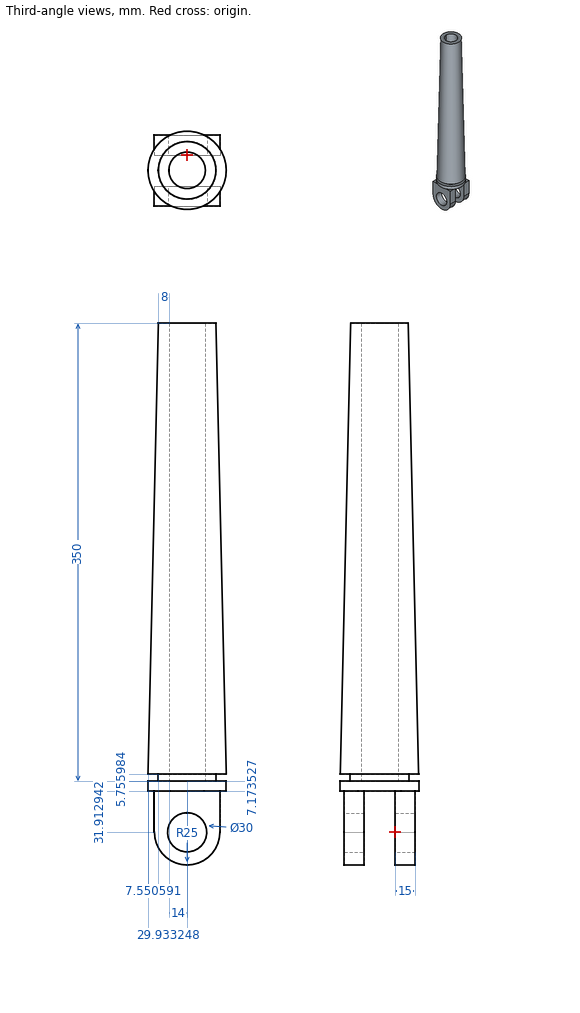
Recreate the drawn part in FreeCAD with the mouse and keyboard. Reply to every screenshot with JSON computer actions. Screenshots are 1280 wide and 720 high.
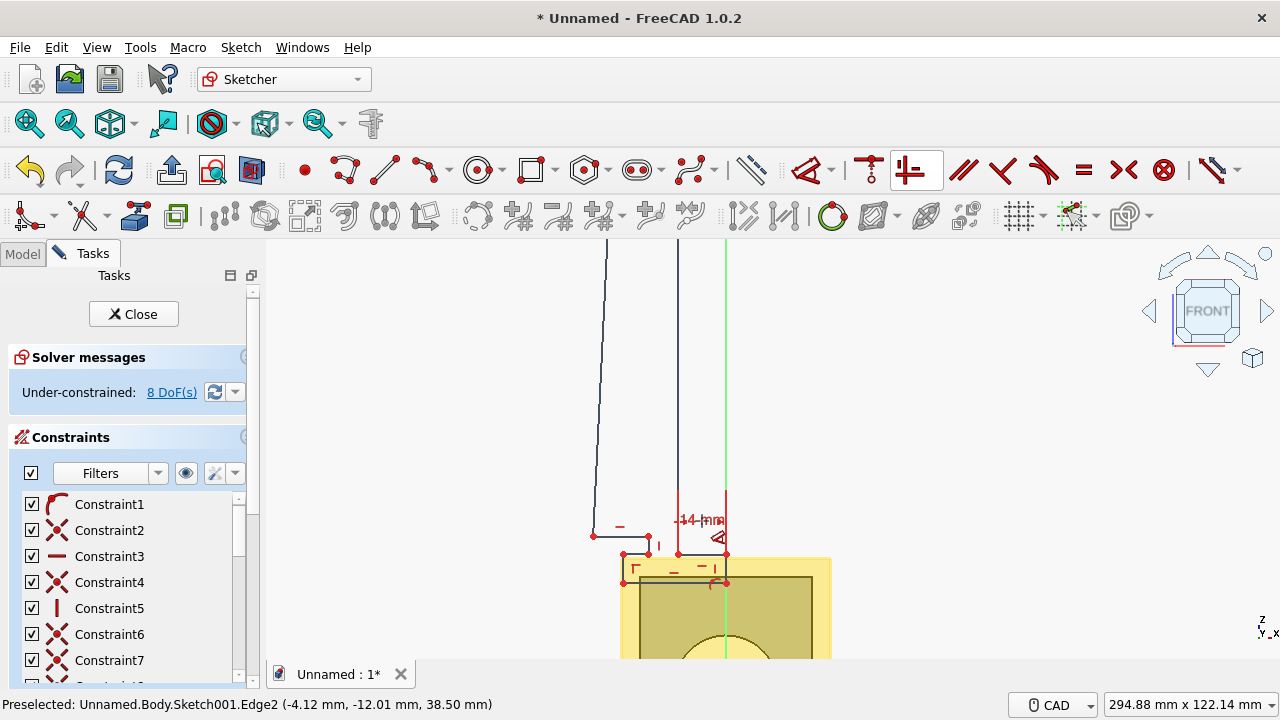
{"action": "scroll", "coordinate": [712, 558], "scroll_direction": "down", "scroll_amount": 8}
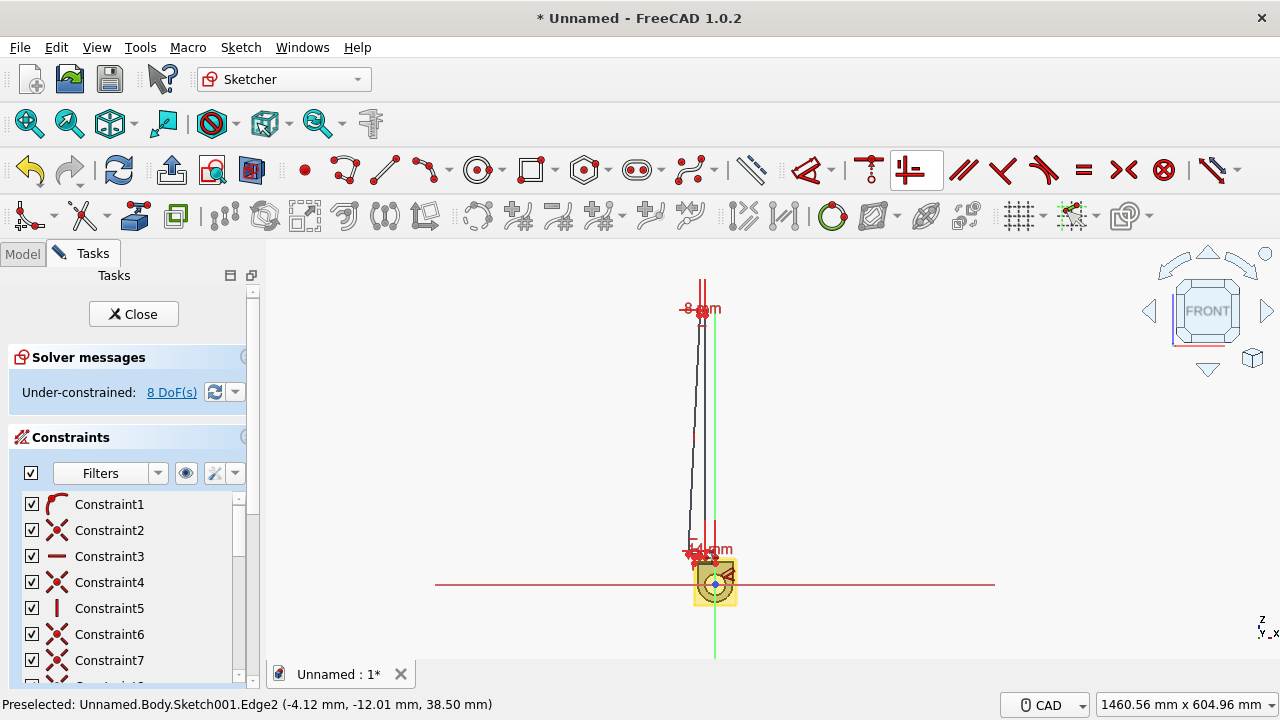
{"action": "scroll", "coordinate": [705, 509], "scroll_direction": "up", "scroll_amount": 2}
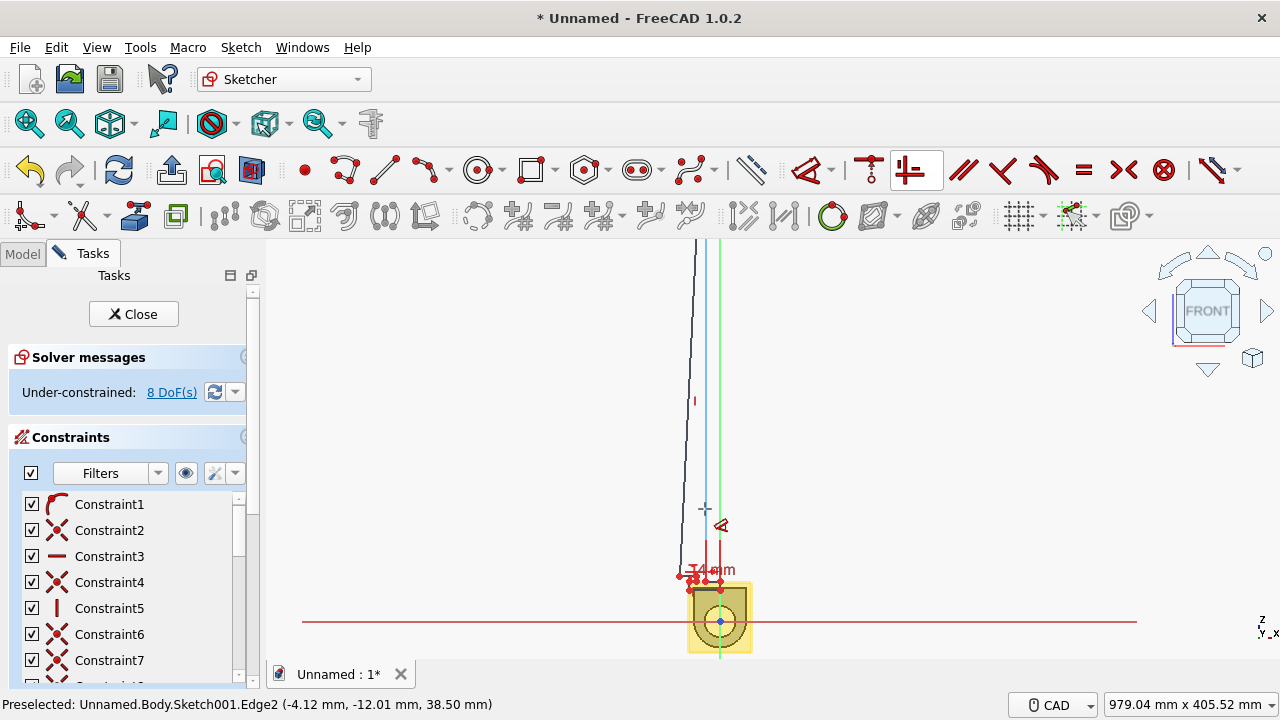
{"action": "left_click", "coordinate": [706, 509]}
{"action": "left_click", "coordinate": [740, 424]}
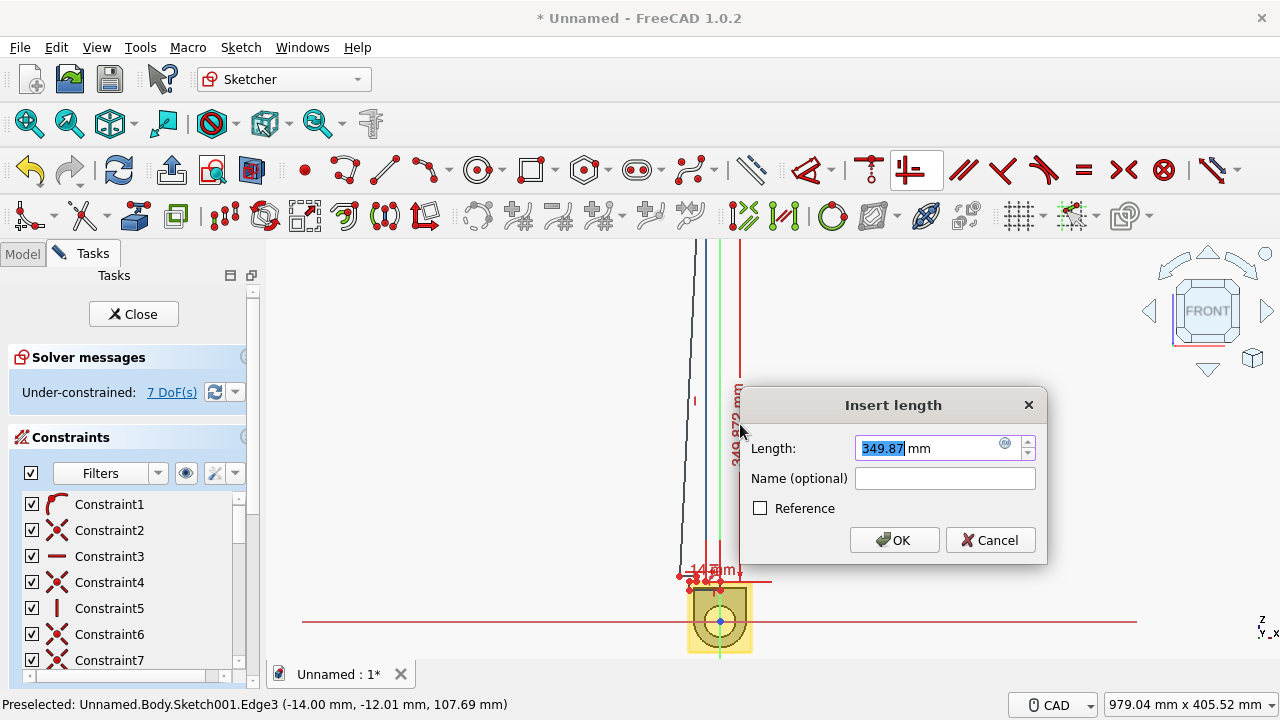
{"action": "type", "text": "350"}
{"action": "key", "text": "Return"}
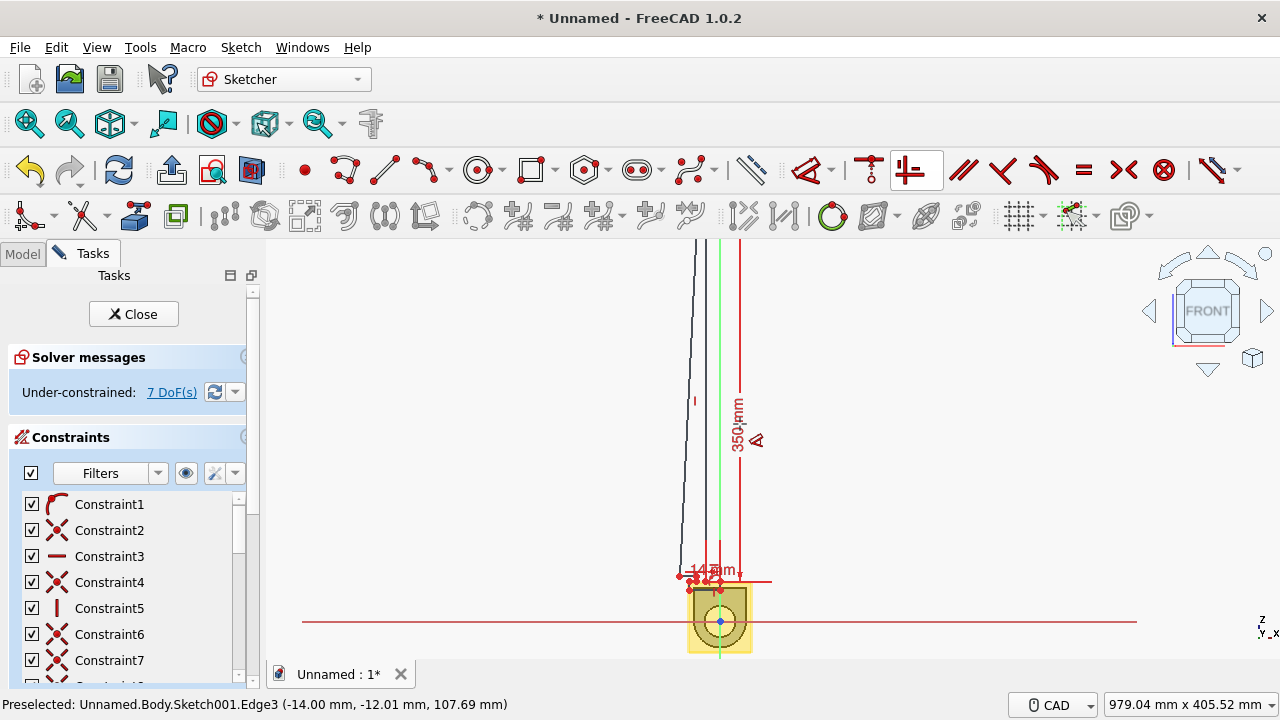
{"action": "scroll", "coordinate": [720, 586], "scroll_direction": "up", "scroll_amount": 9}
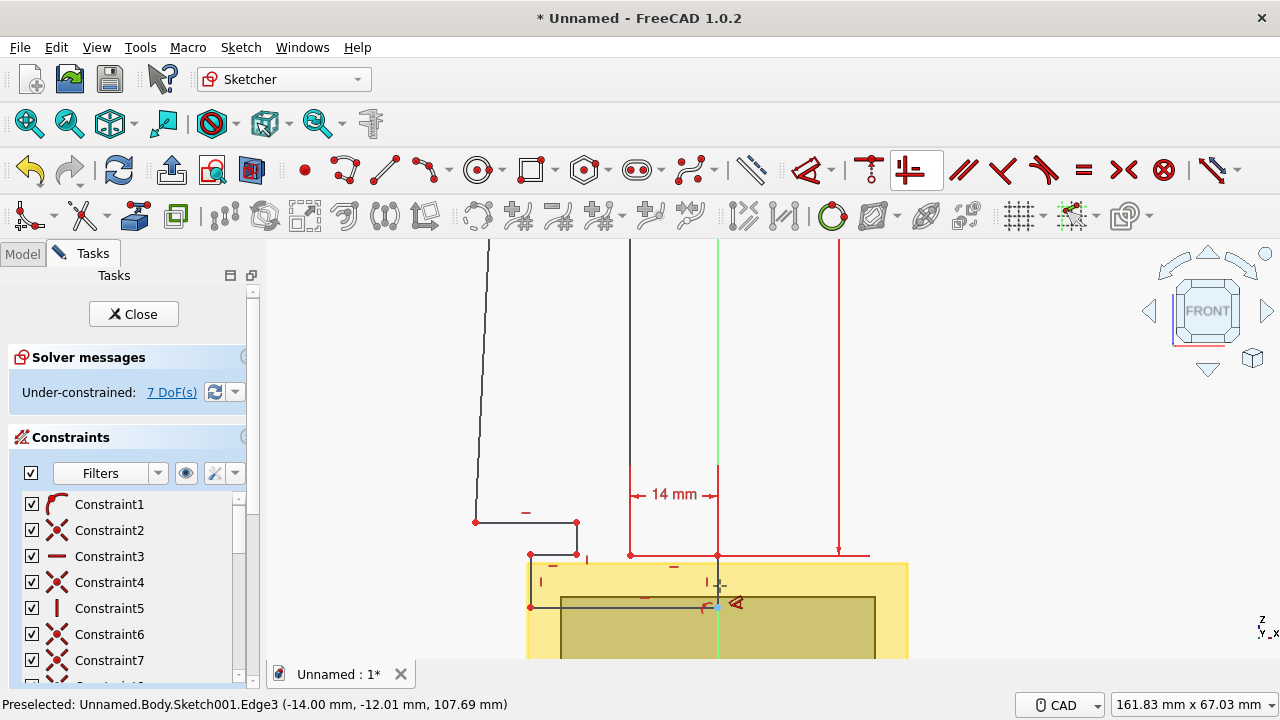
{"action": "left_click", "coordinate": [718, 582]}
{"action": "left_click", "coordinate": [752, 582]}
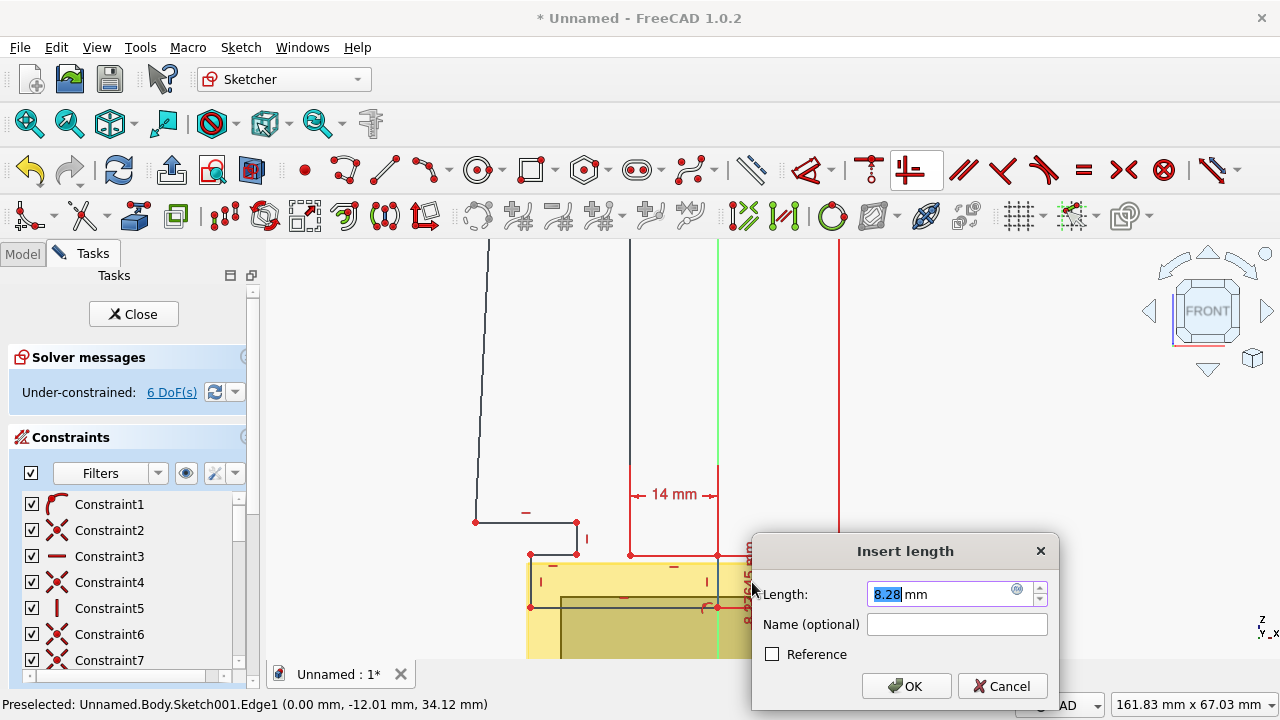
{"action": "type", "text": "7.173527"}
{"action": "key", "text": "Return"}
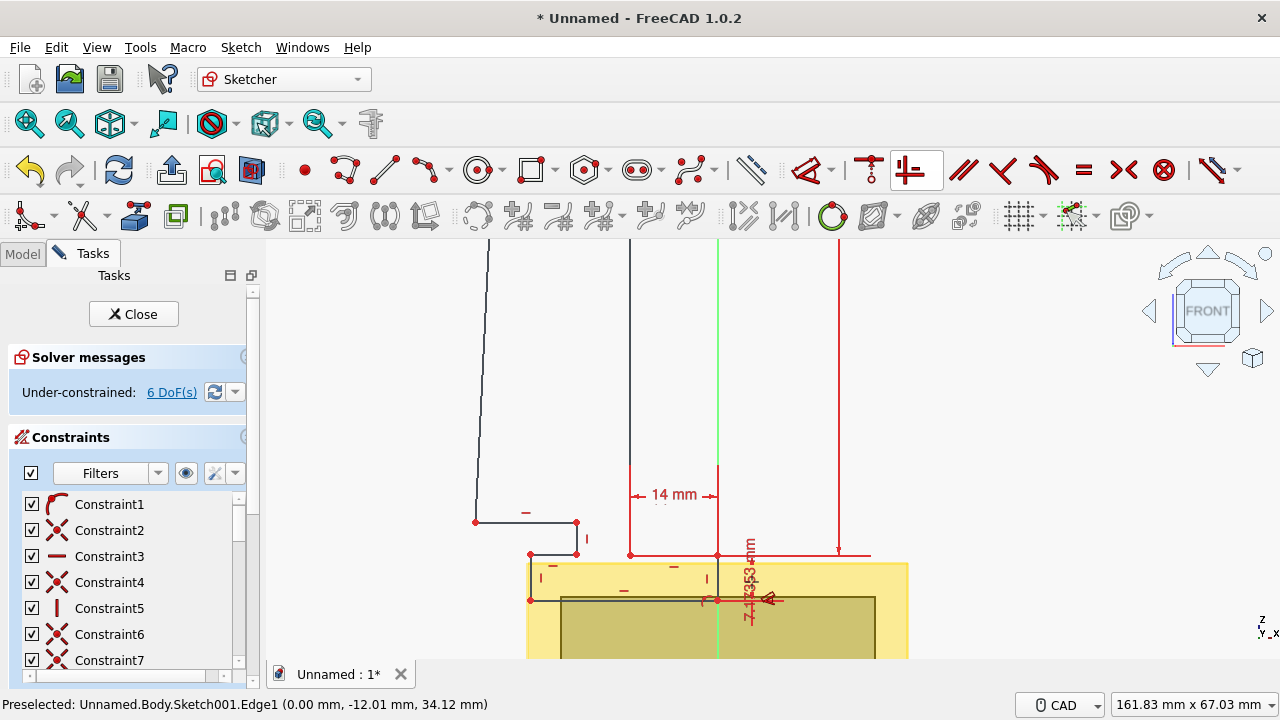
{"action": "left_click", "coordinate": [506, 523]}
{"action": "left_click", "coordinate": [503, 557]}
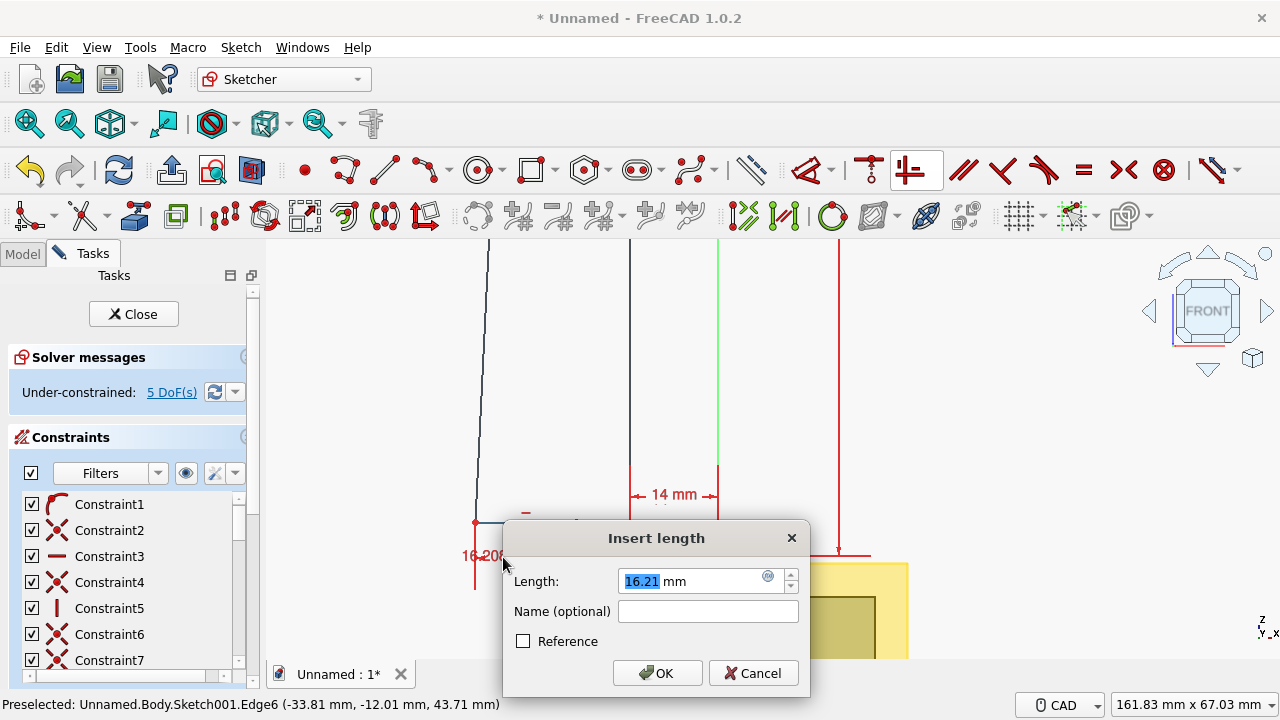
{"action": "type", "text": "7.550591"}
{"action": "key", "text": "Return"}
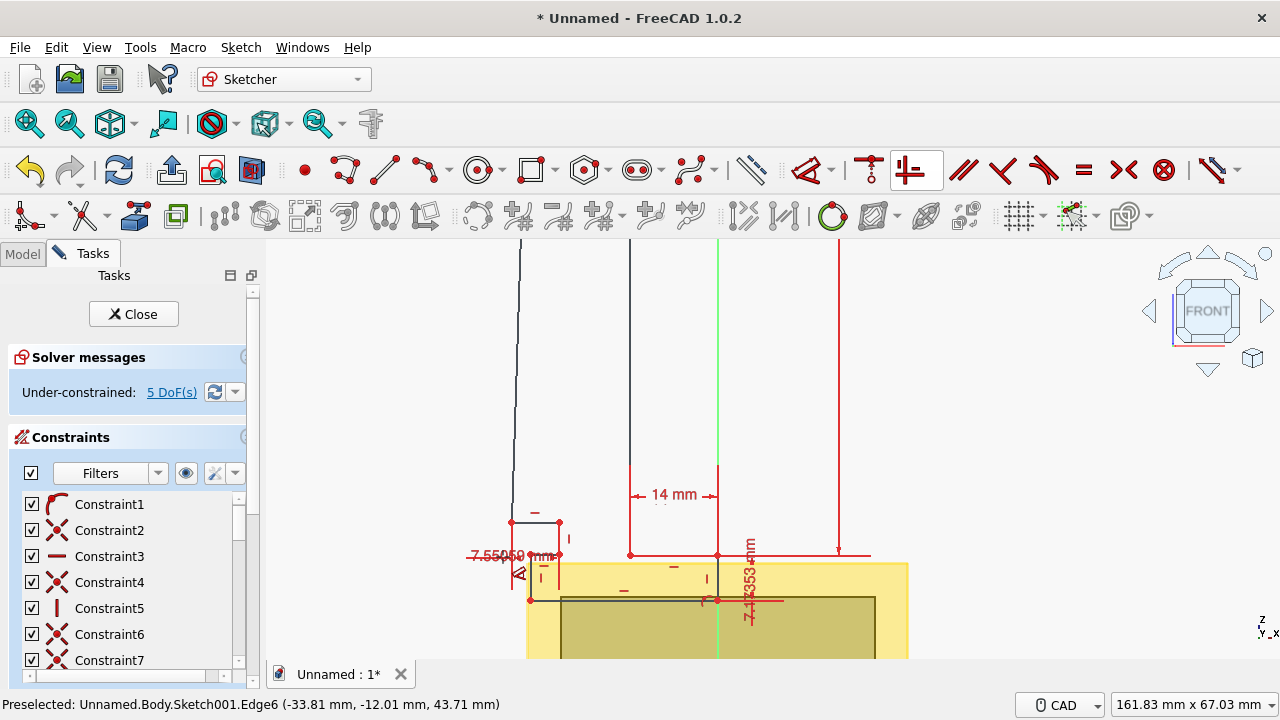
{"action": "scroll", "coordinate": [559, 532], "scroll_direction": "up", "scroll_amount": 2}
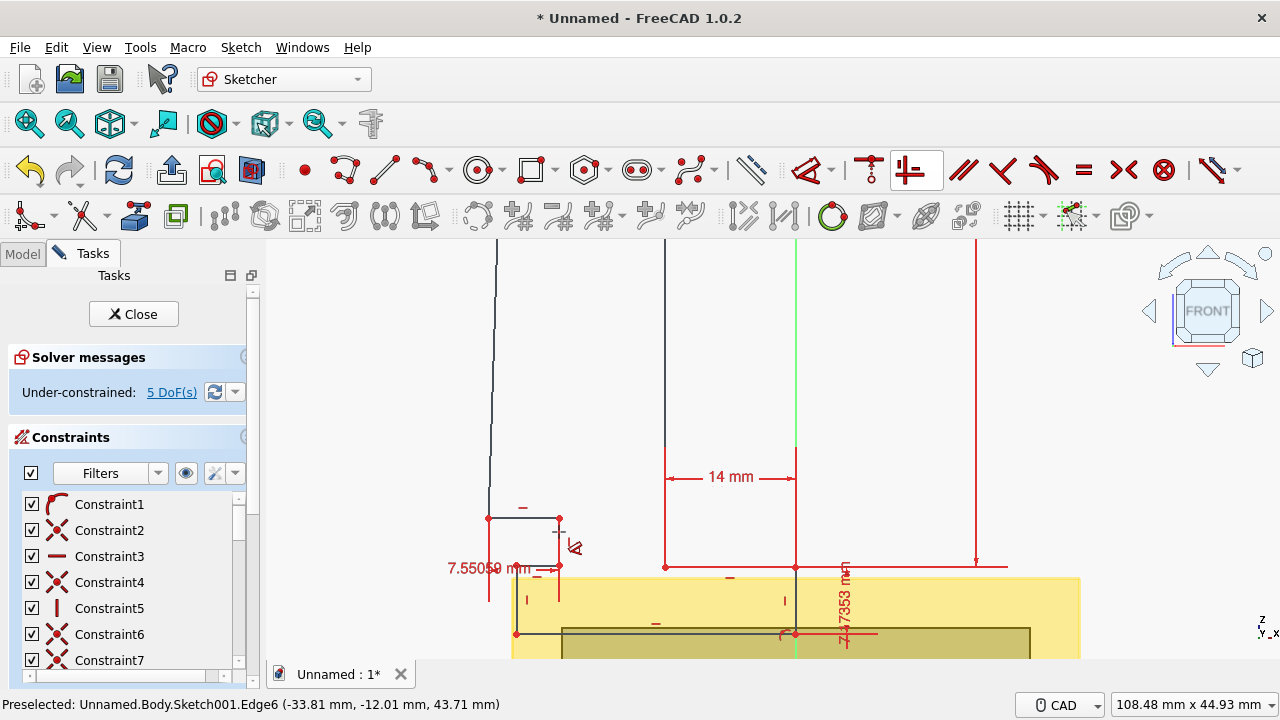
{"action": "left_click", "coordinate": [559, 532]}
{"action": "left_click", "coordinate": [525, 542]}